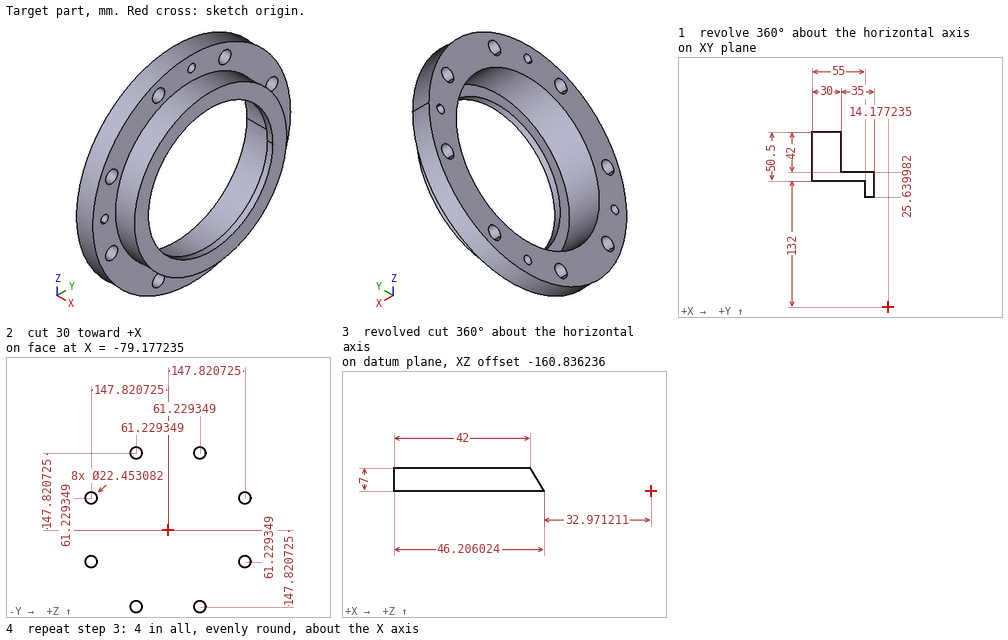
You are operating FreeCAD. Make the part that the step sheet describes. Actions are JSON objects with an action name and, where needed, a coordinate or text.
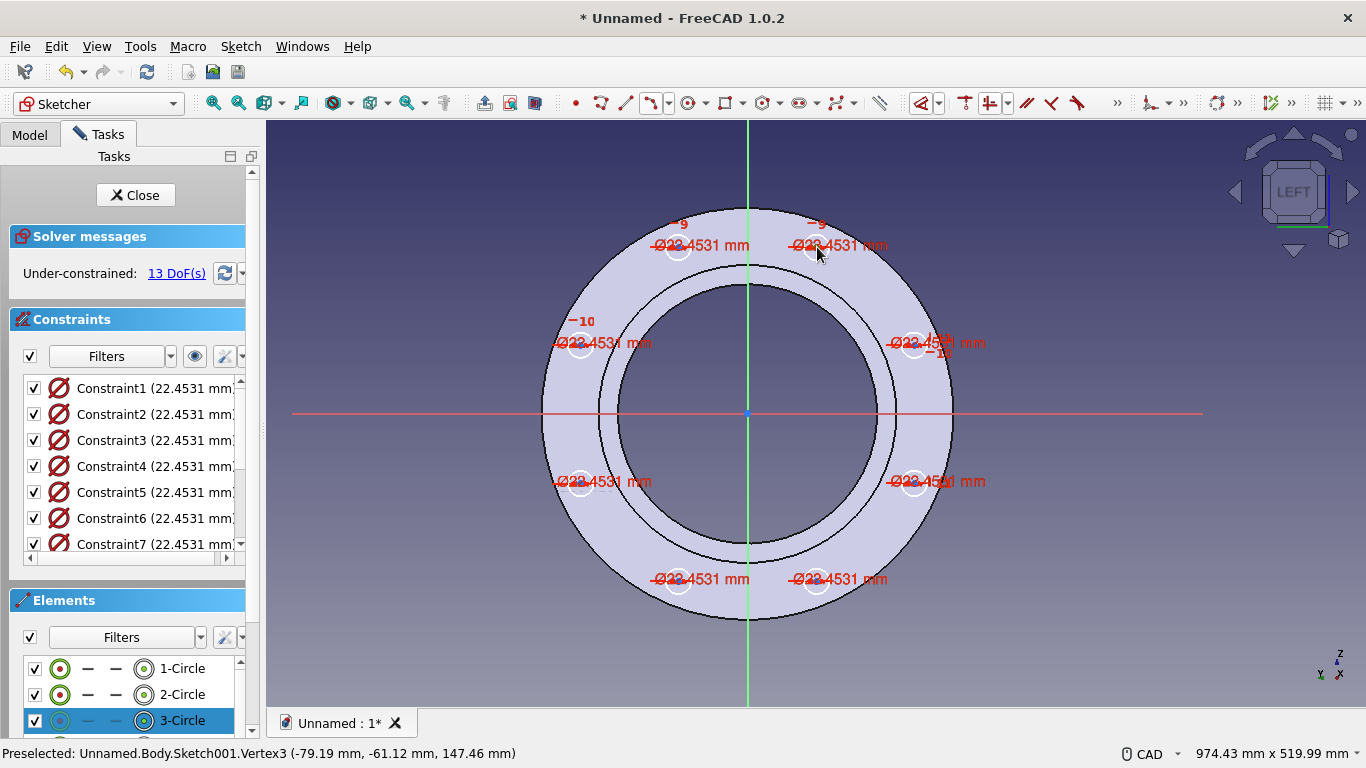
{"action": "left_click", "coordinate": [817, 581]}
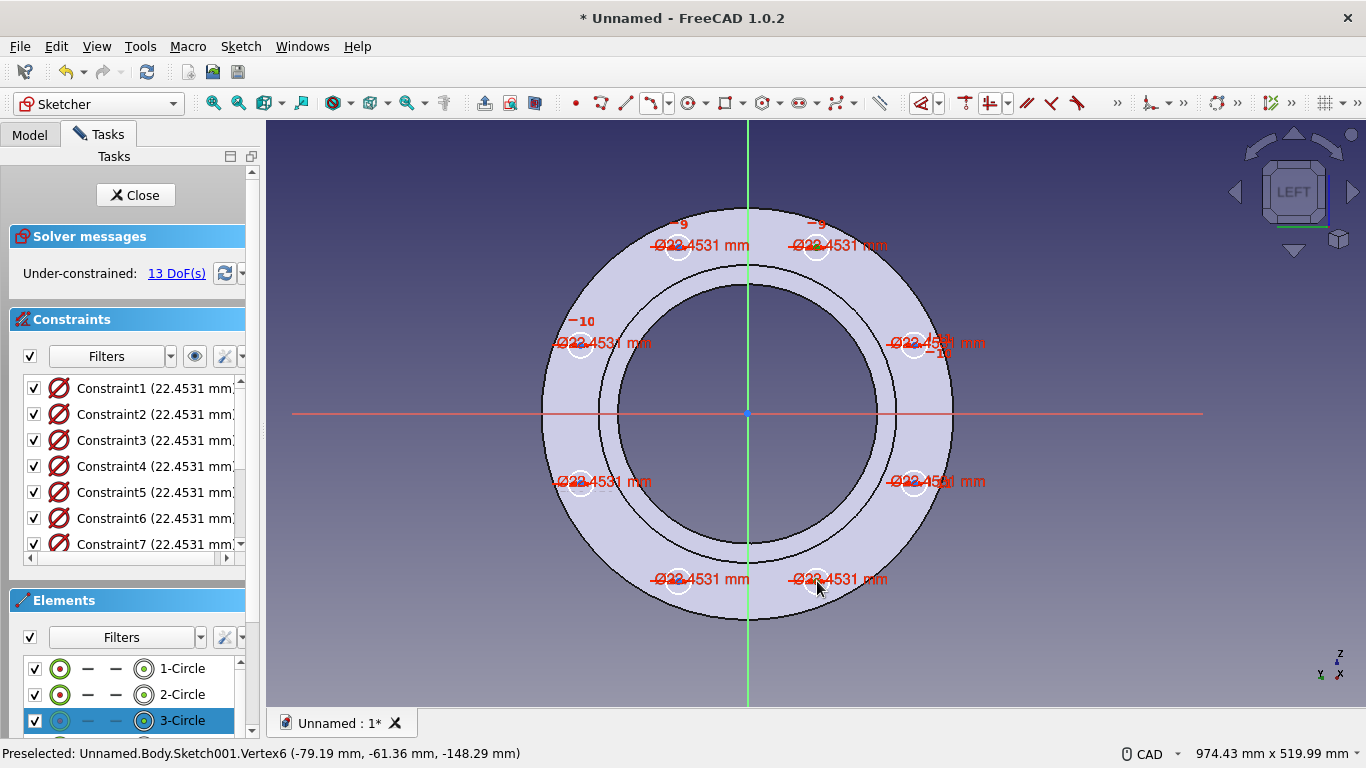
{"action": "left_click", "coordinate": [1008, 104]}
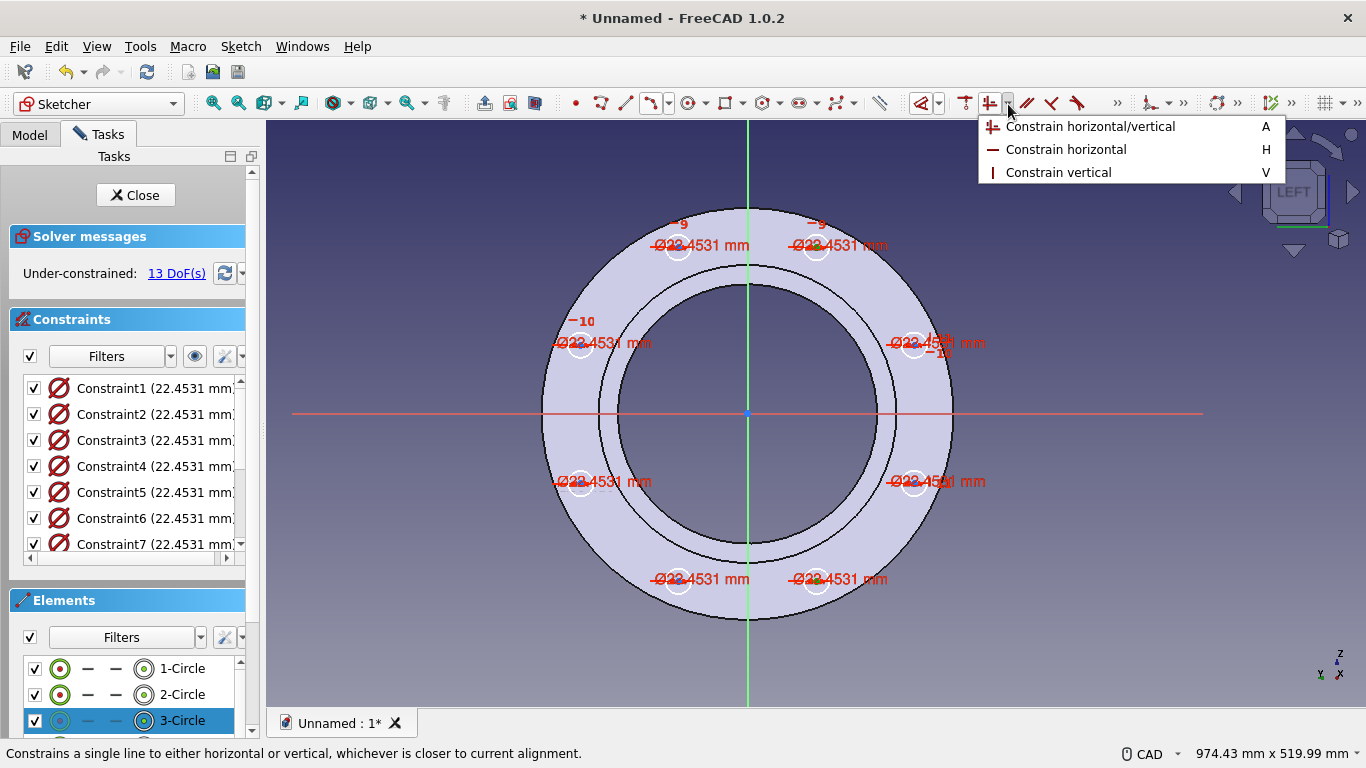
{"action": "left_click", "coordinate": [1132, 172]}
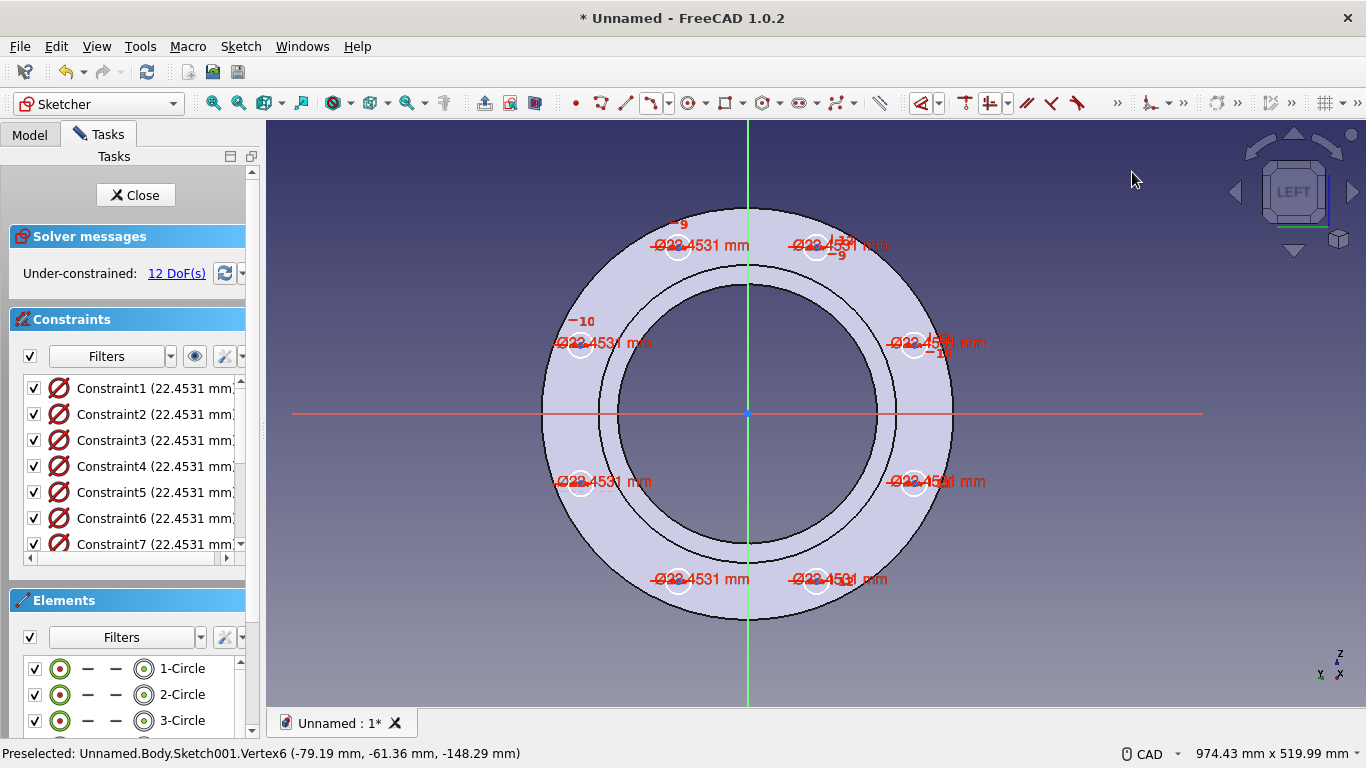
{"action": "left_click", "coordinate": [678, 247]}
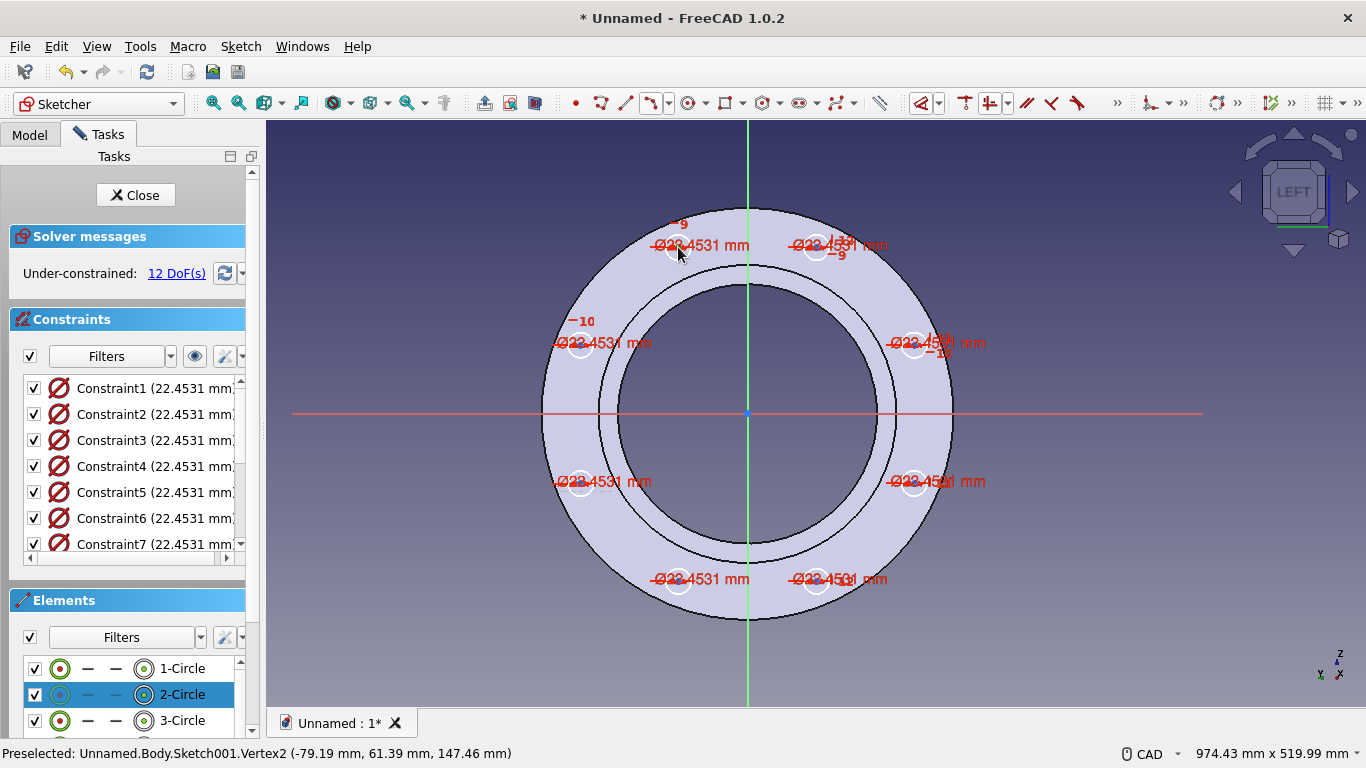
{"action": "left_click", "coordinate": [678, 581]}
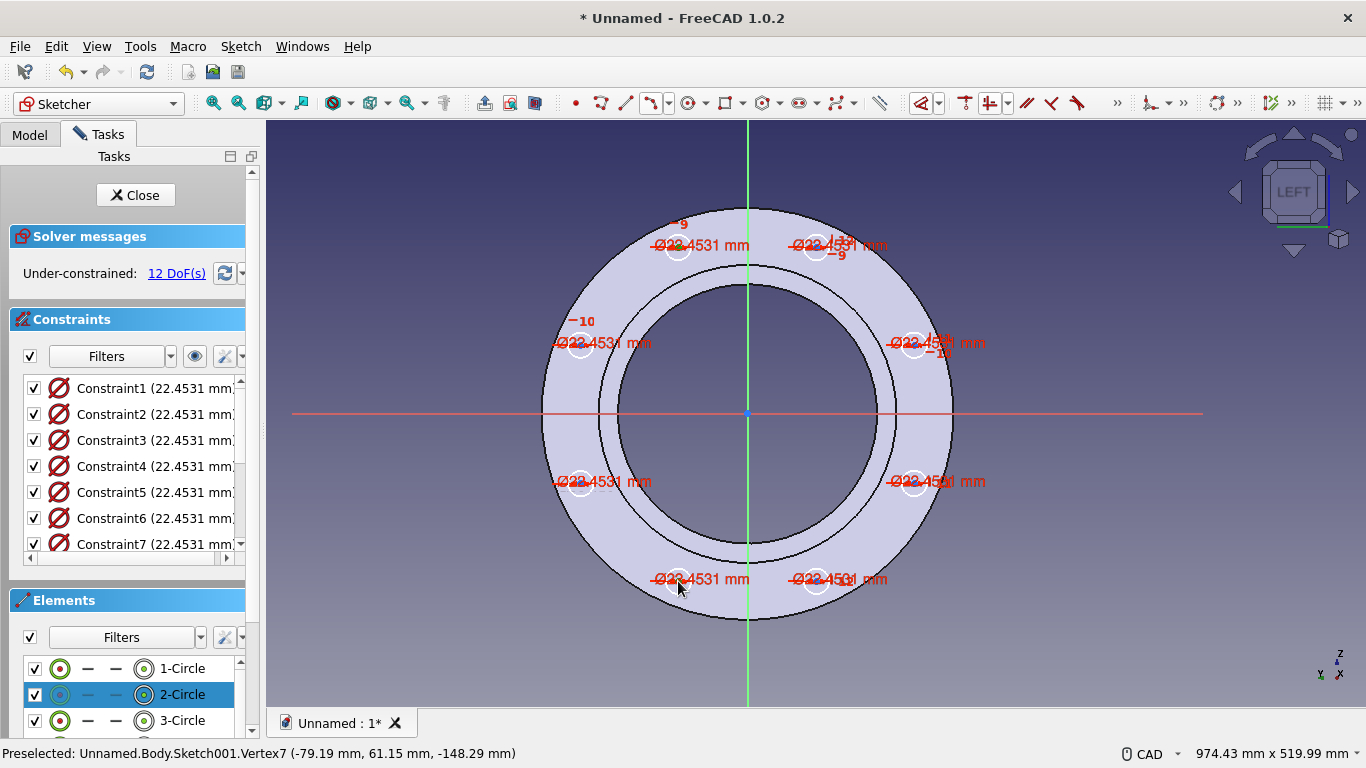
{"action": "left_click", "coordinate": [1008, 104]}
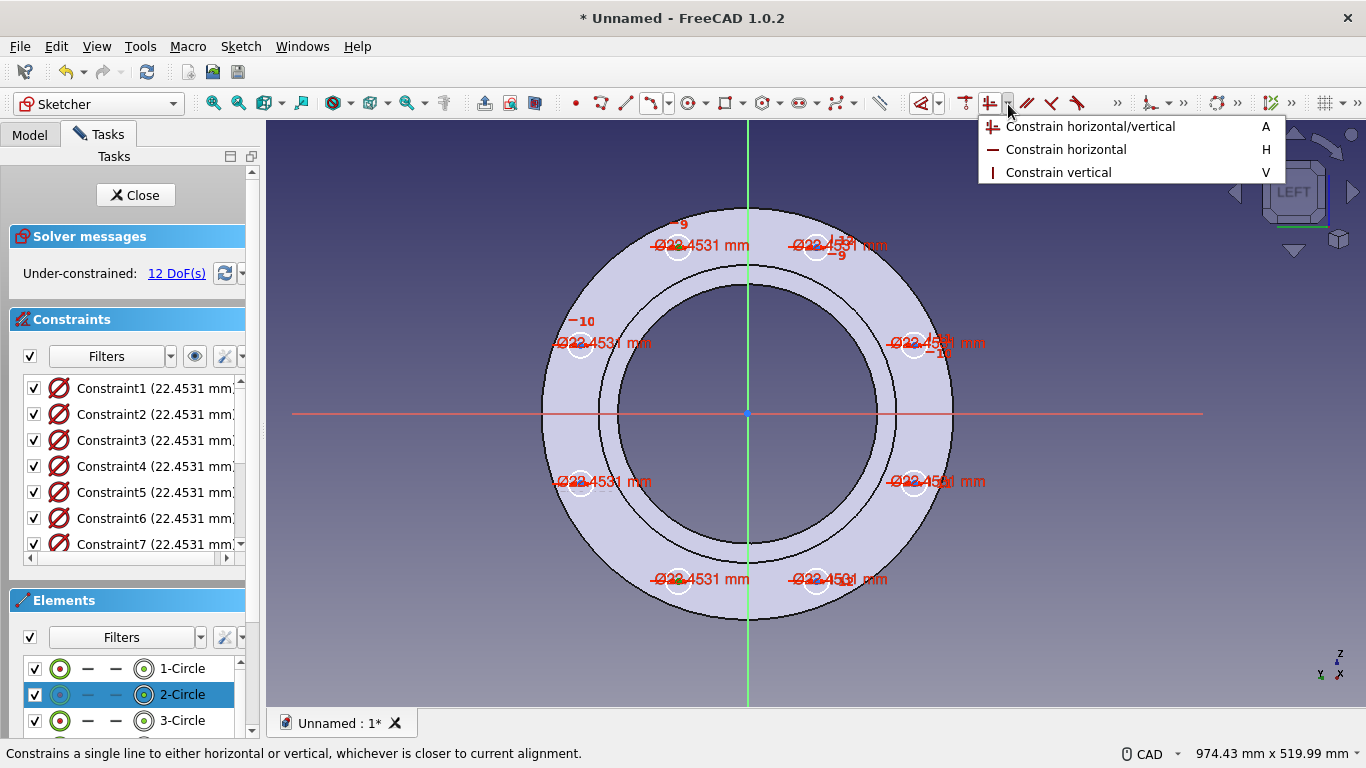
{"action": "left_click", "coordinate": [1132, 172]}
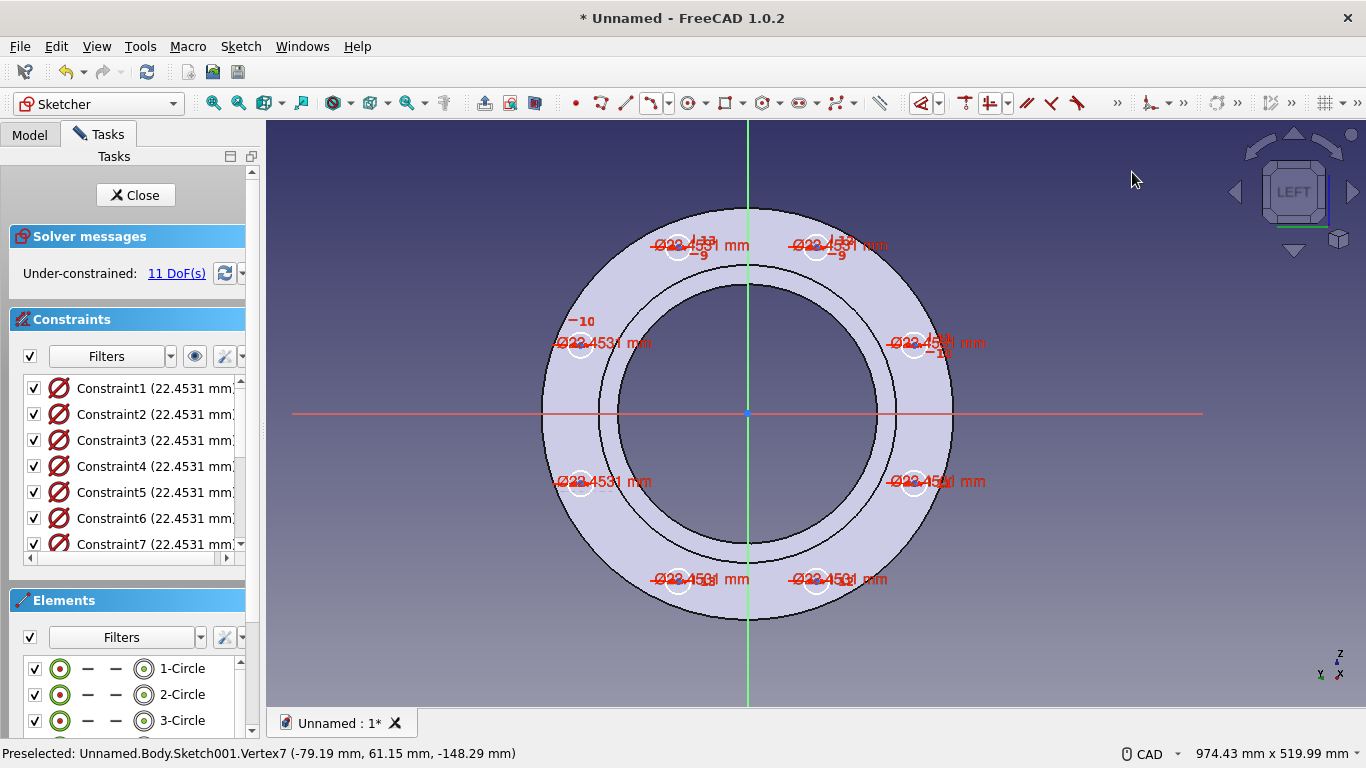
{"action": "left_click", "coordinate": [817, 581]}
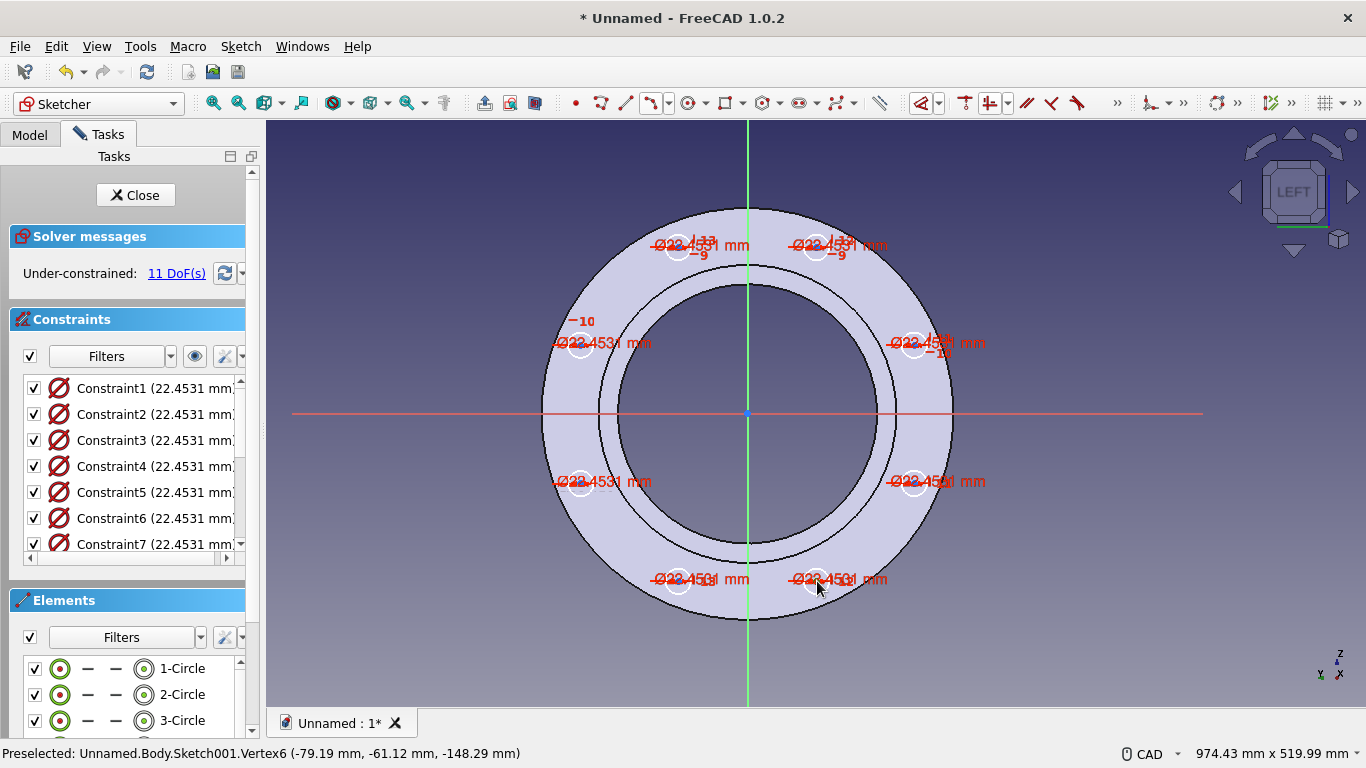
{"action": "left_click", "coordinate": [678, 581]}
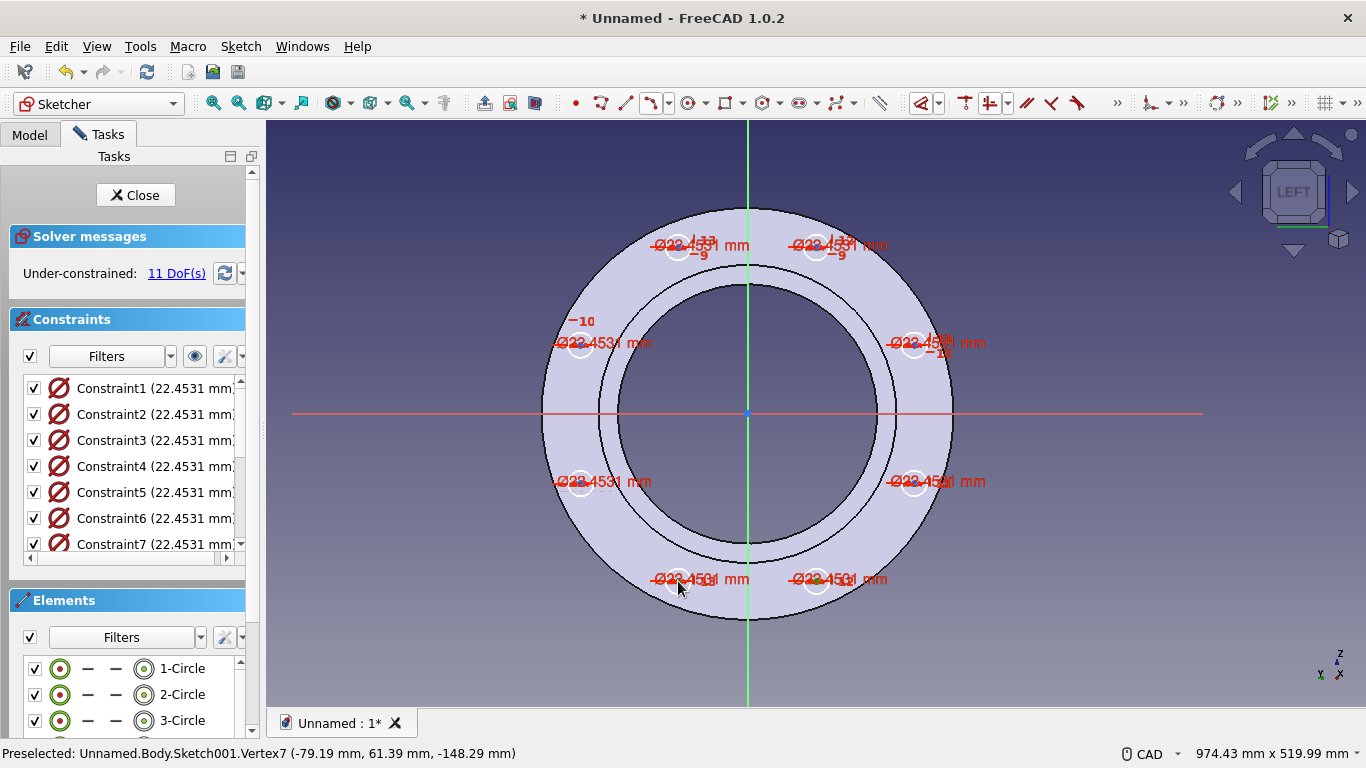
{"action": "key", "text": "h"}